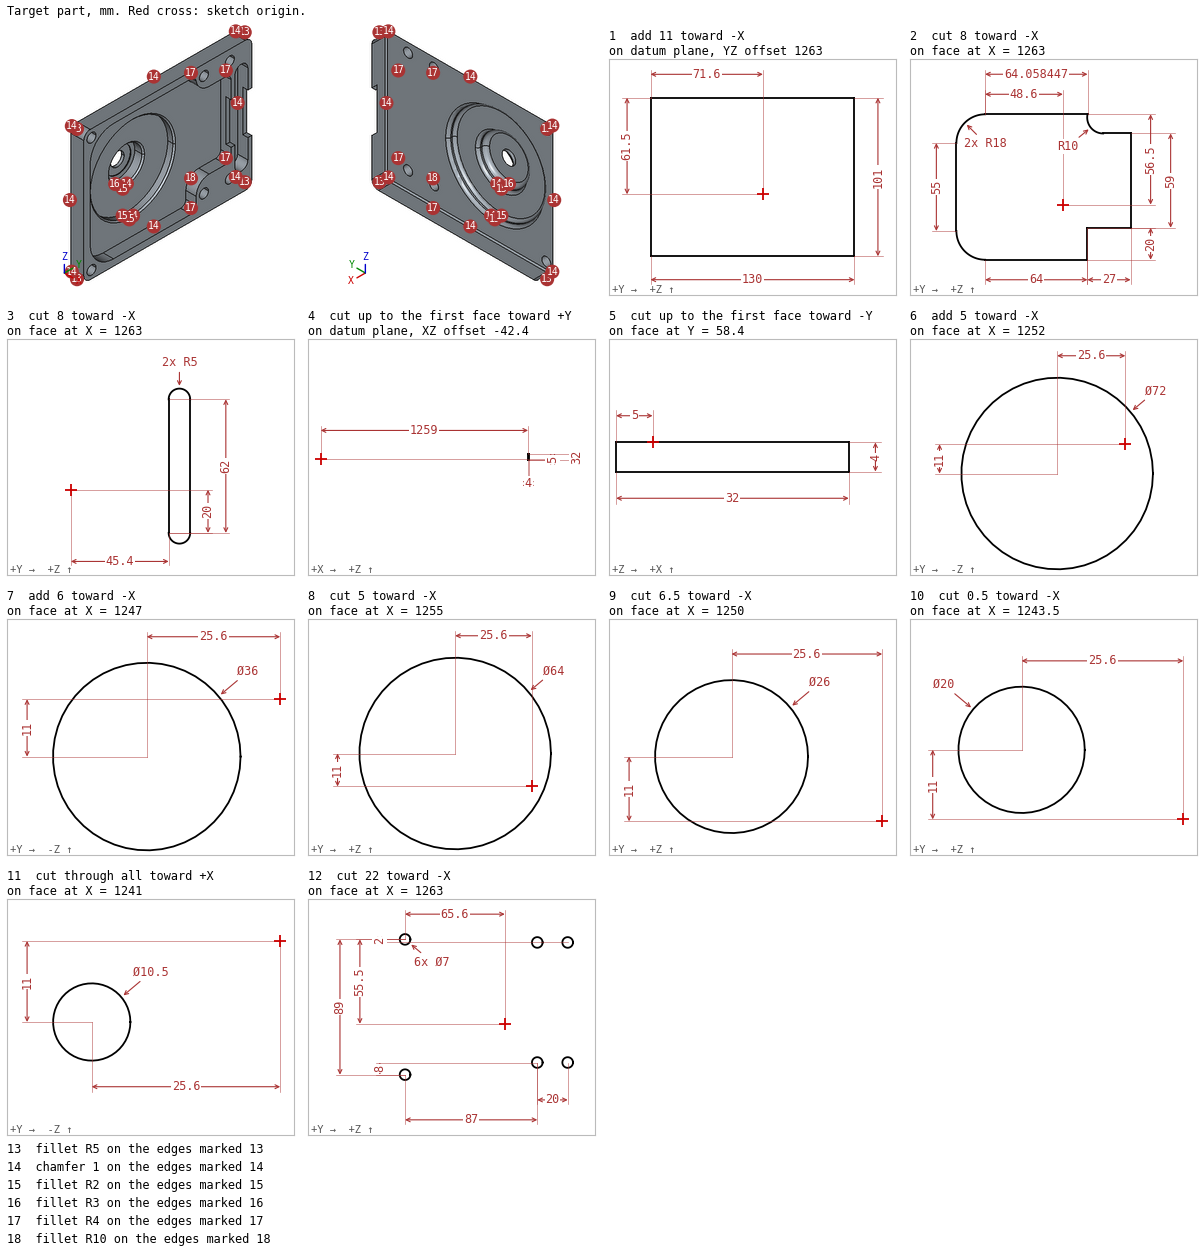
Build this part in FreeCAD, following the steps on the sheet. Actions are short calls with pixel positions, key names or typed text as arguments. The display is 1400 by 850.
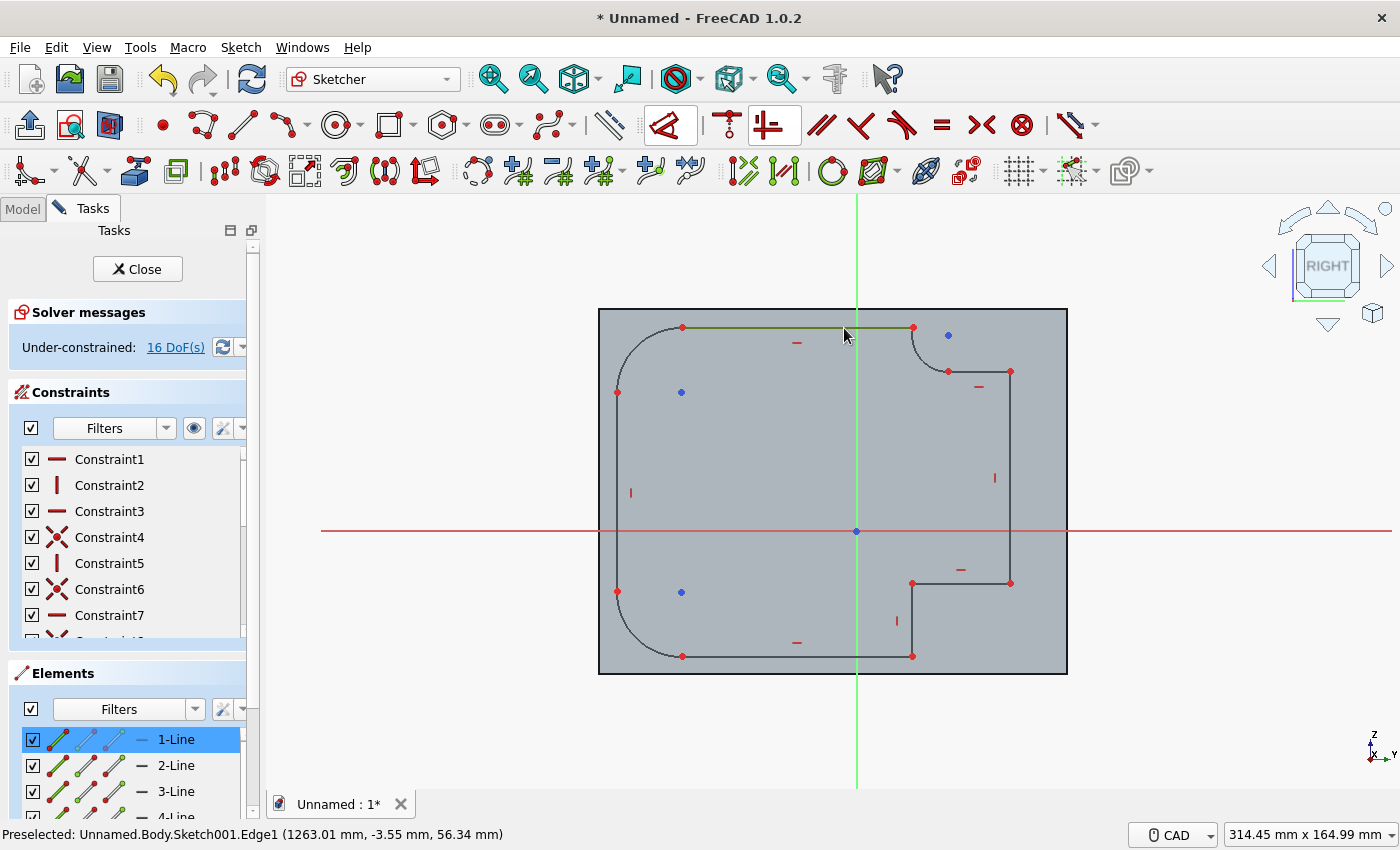
click(652, 335)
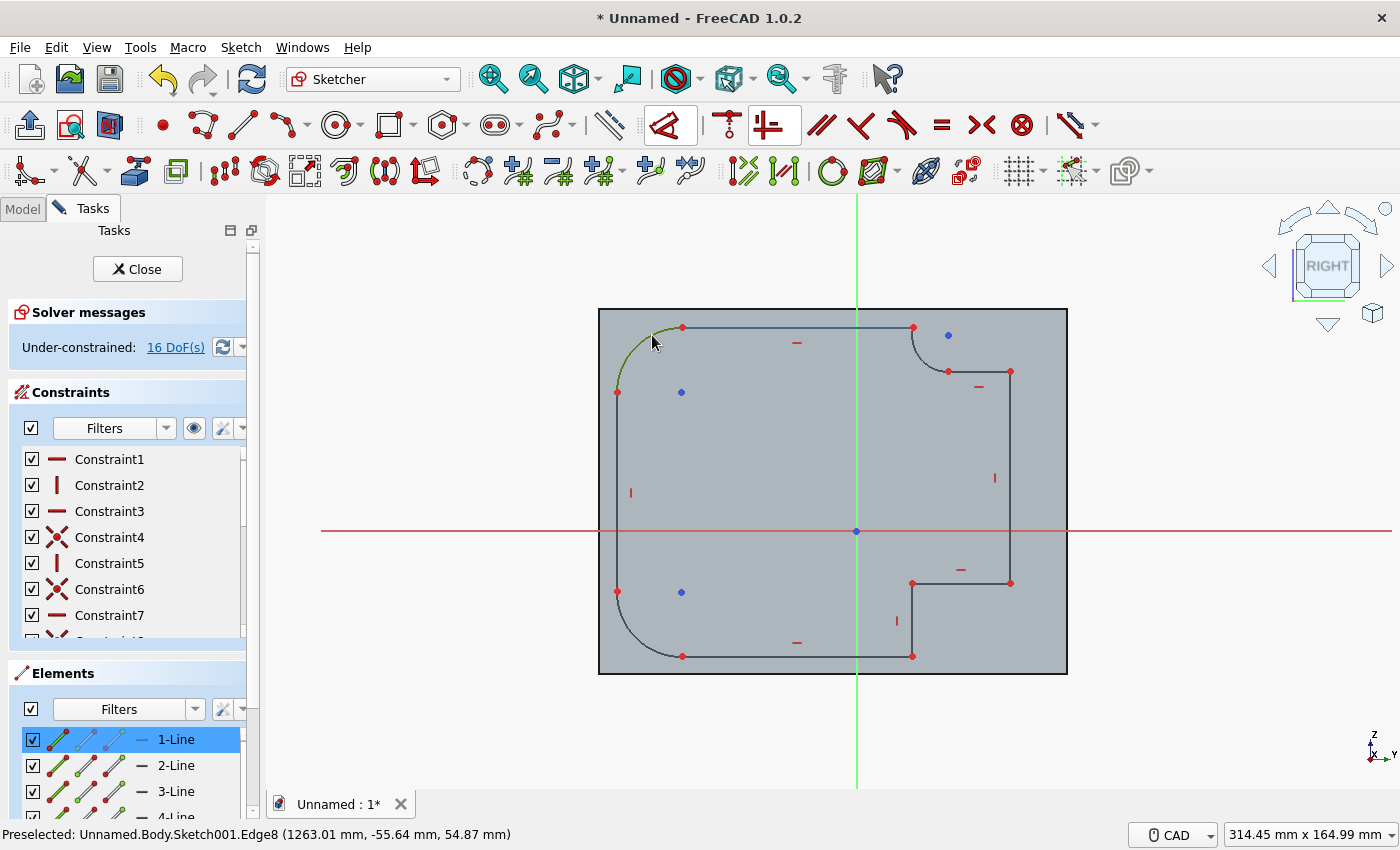
key(t)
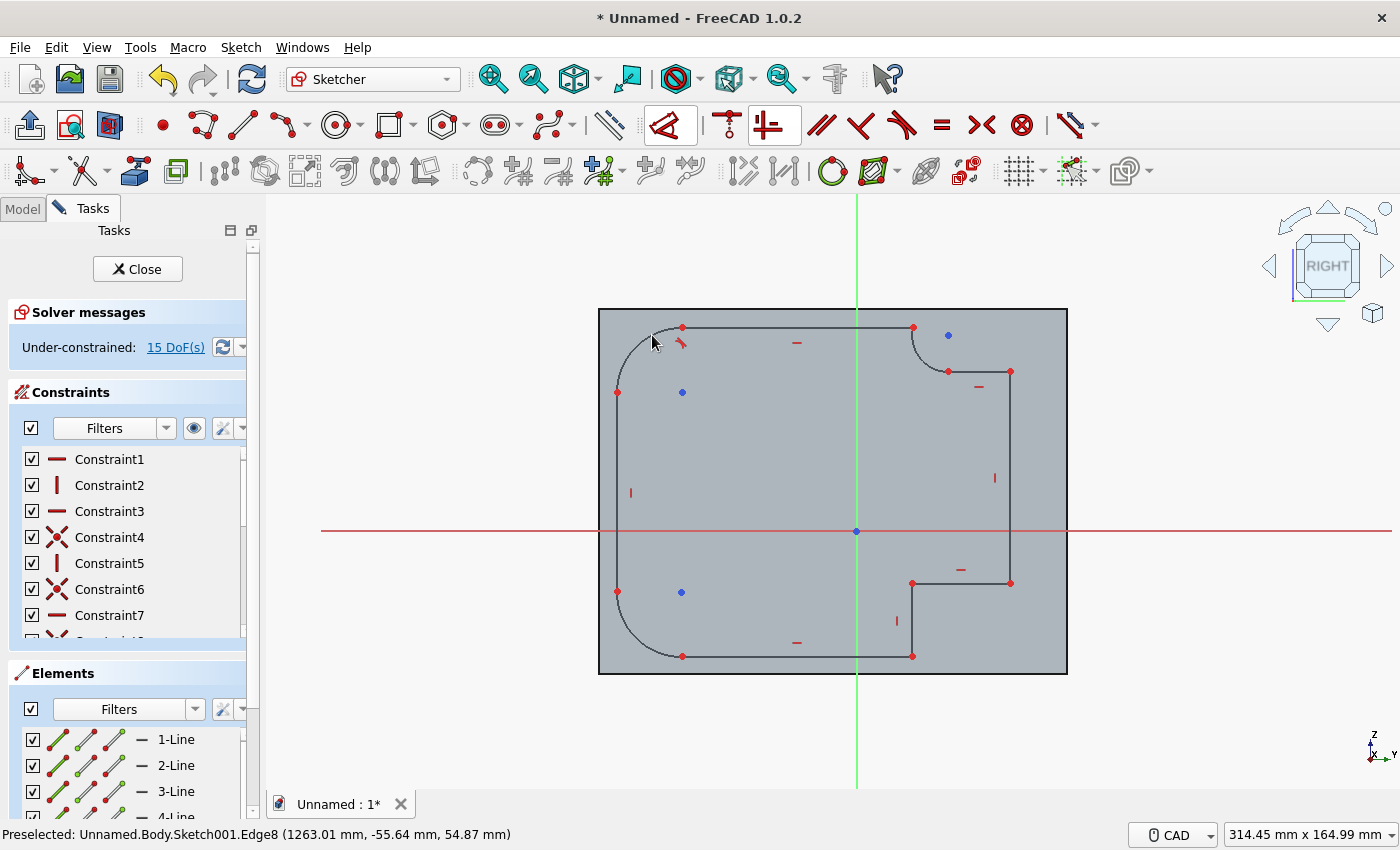
click(617, 453)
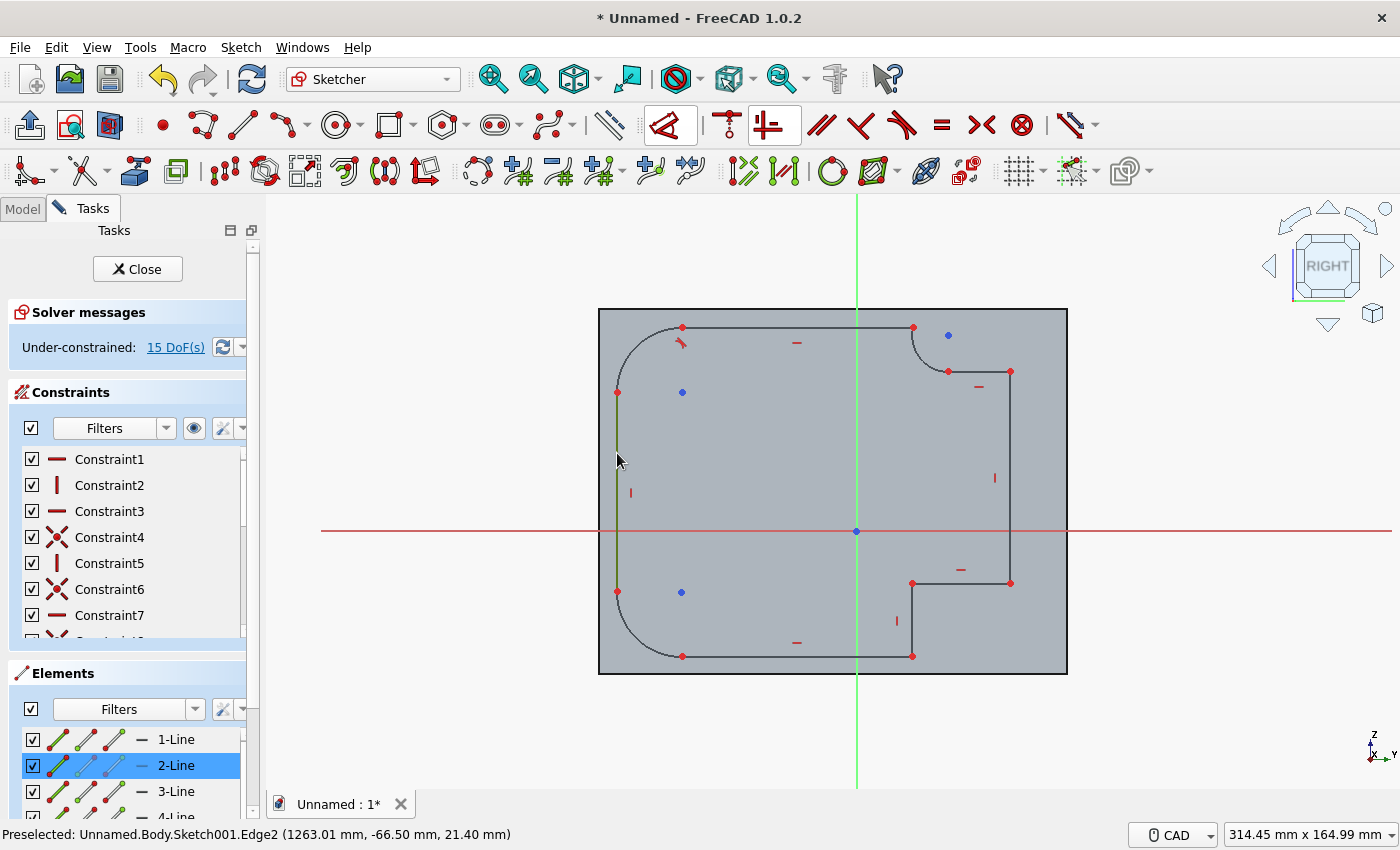
click(652, 335)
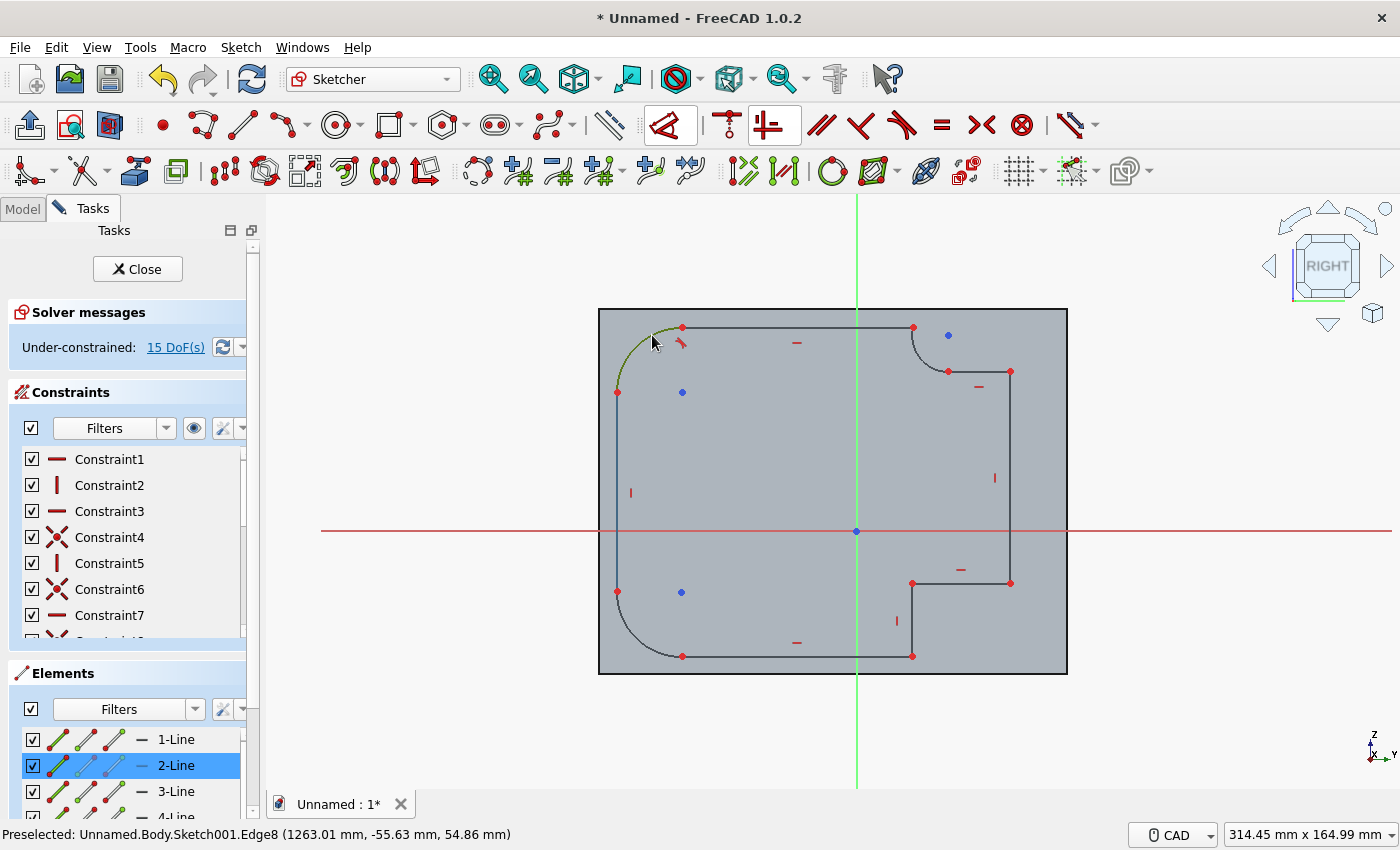
key(t)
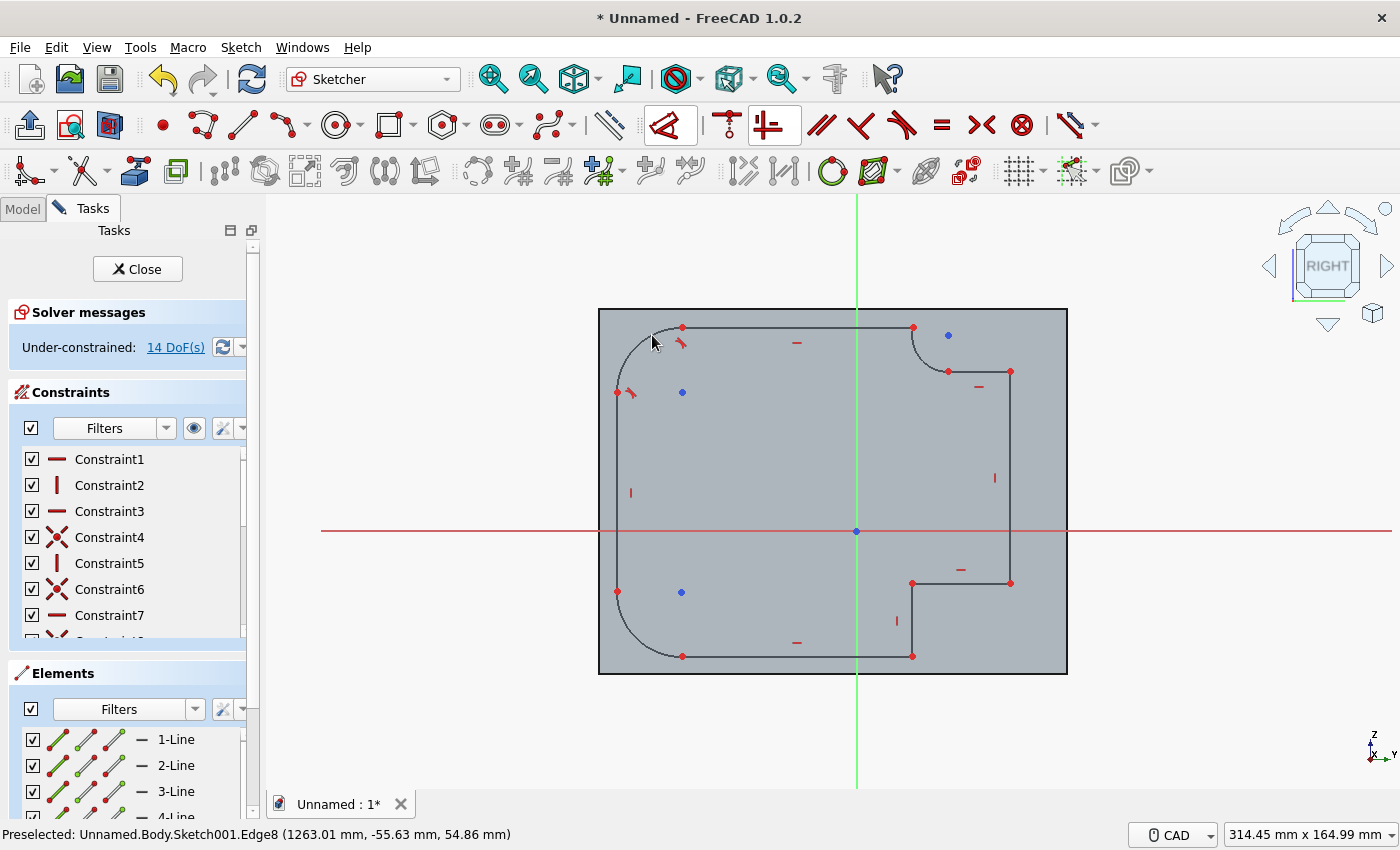
click(617, 453)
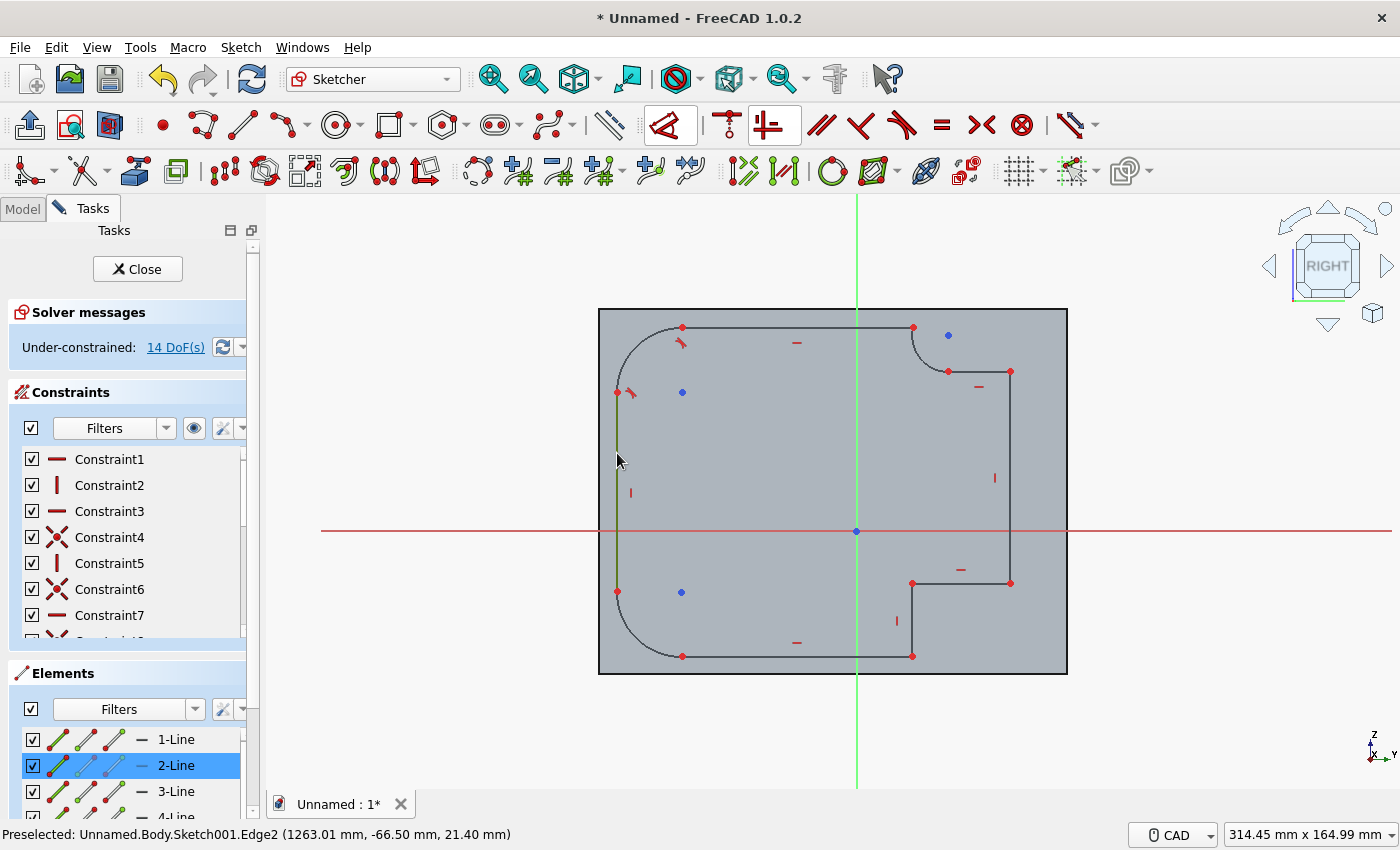
click(624, 622)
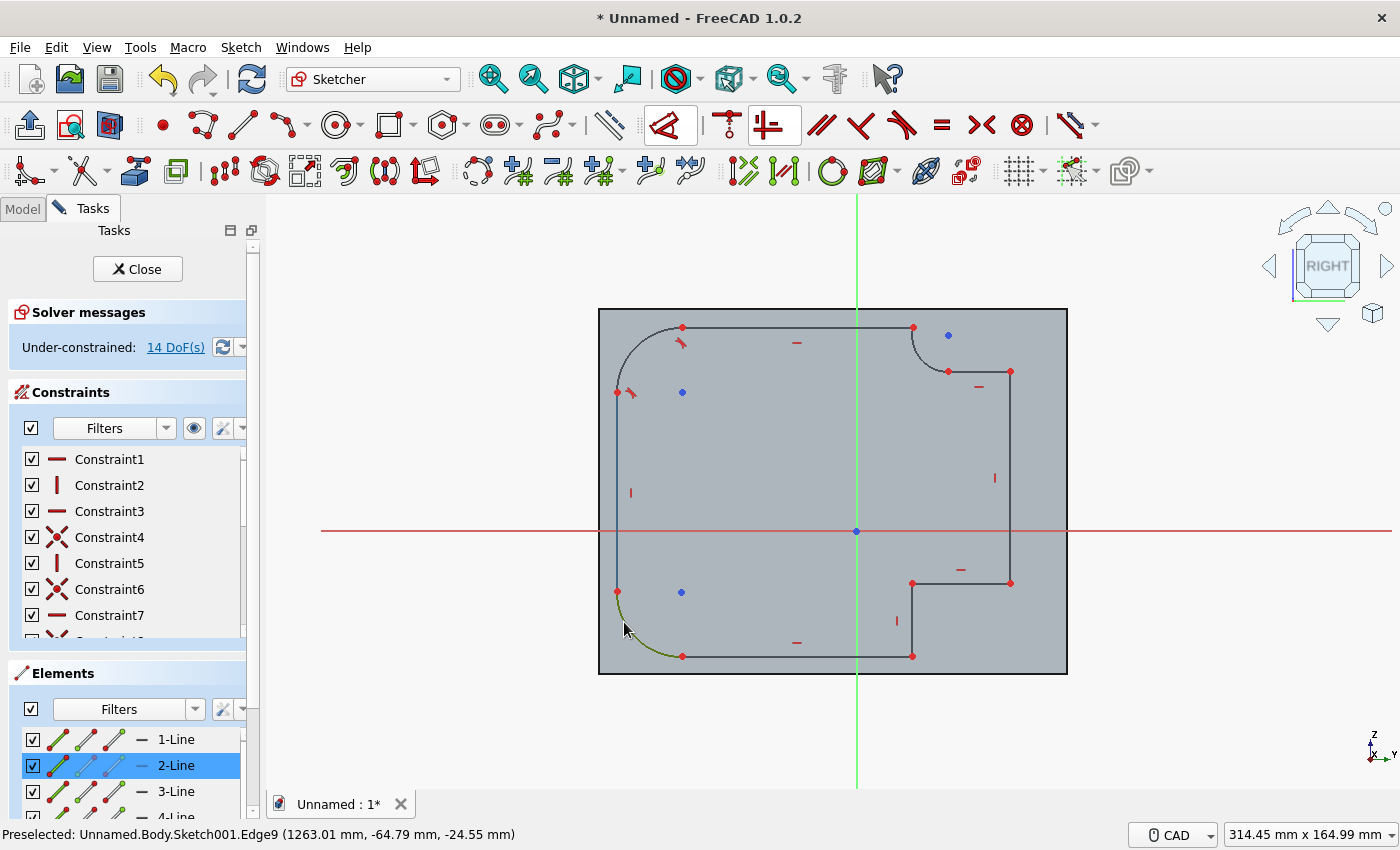
key(t)